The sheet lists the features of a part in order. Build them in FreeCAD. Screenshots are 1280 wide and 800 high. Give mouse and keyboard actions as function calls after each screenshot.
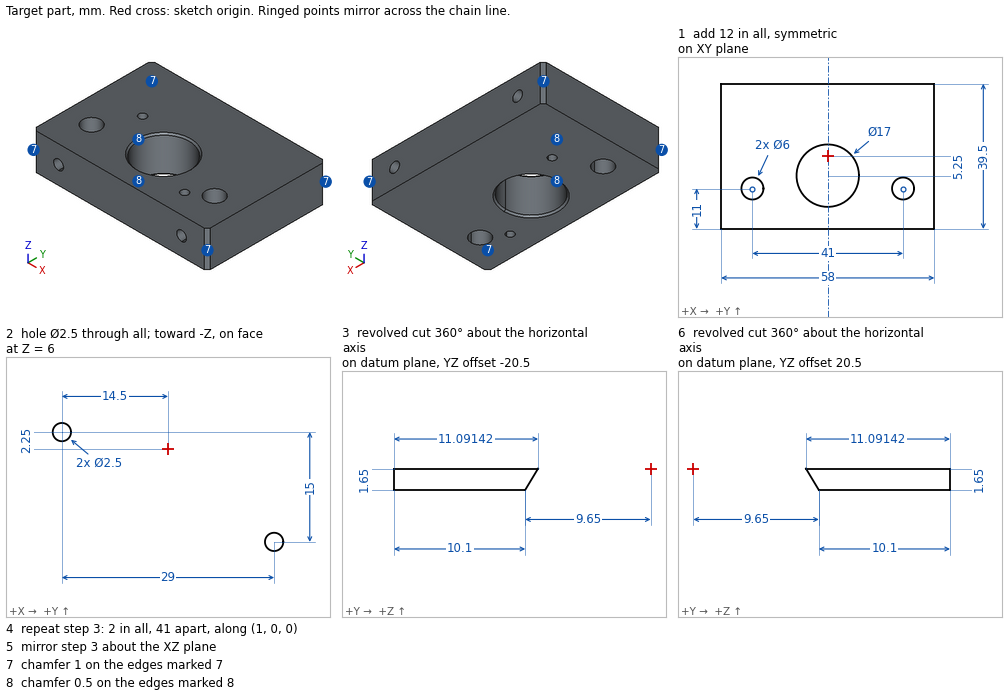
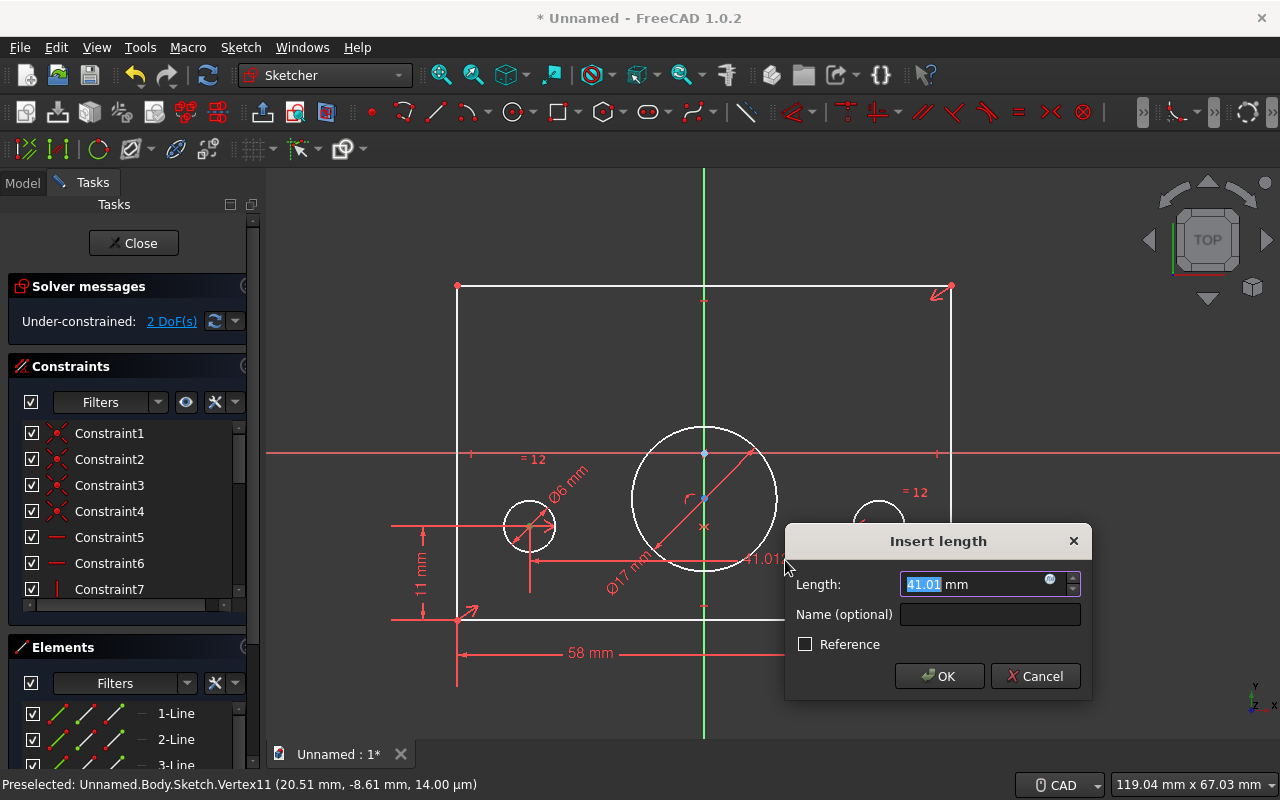
text(41)
key(Return)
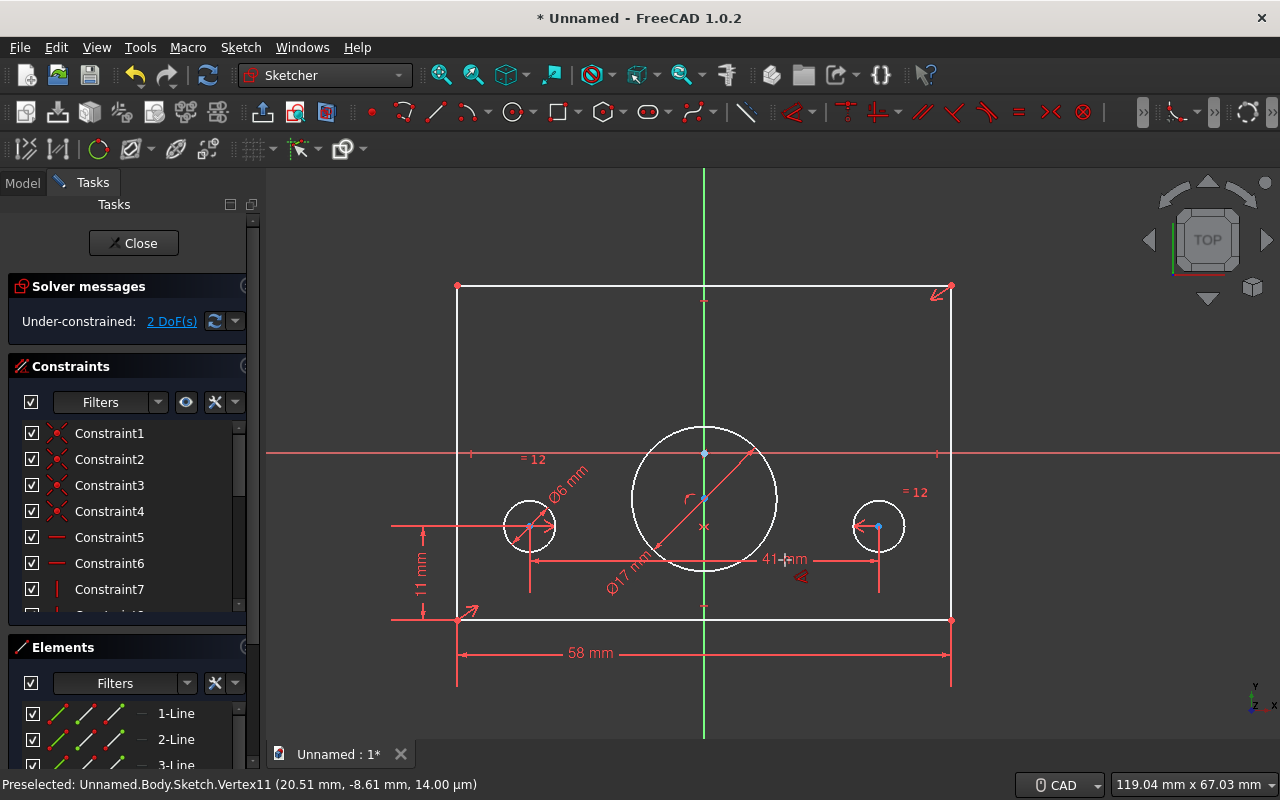
click(951, 520)
click(985, 376)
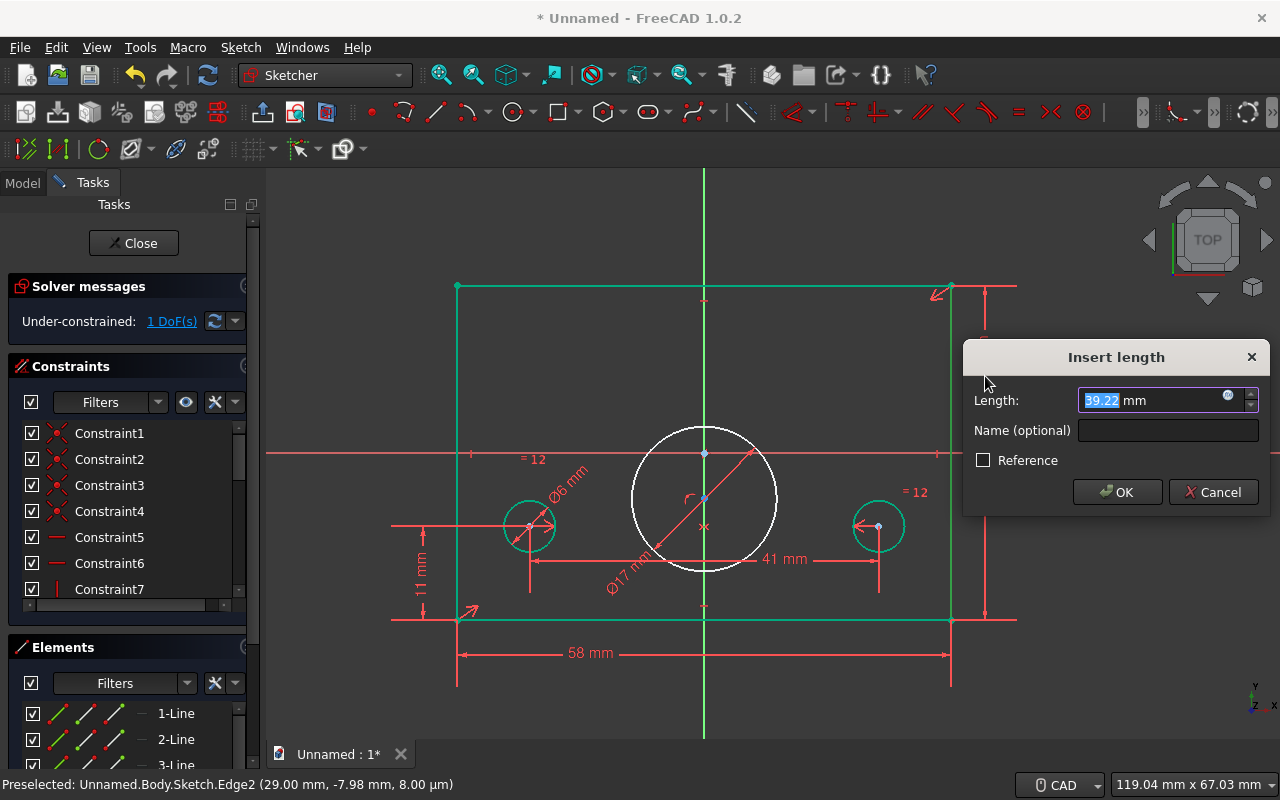
text(39.5)
key(Return)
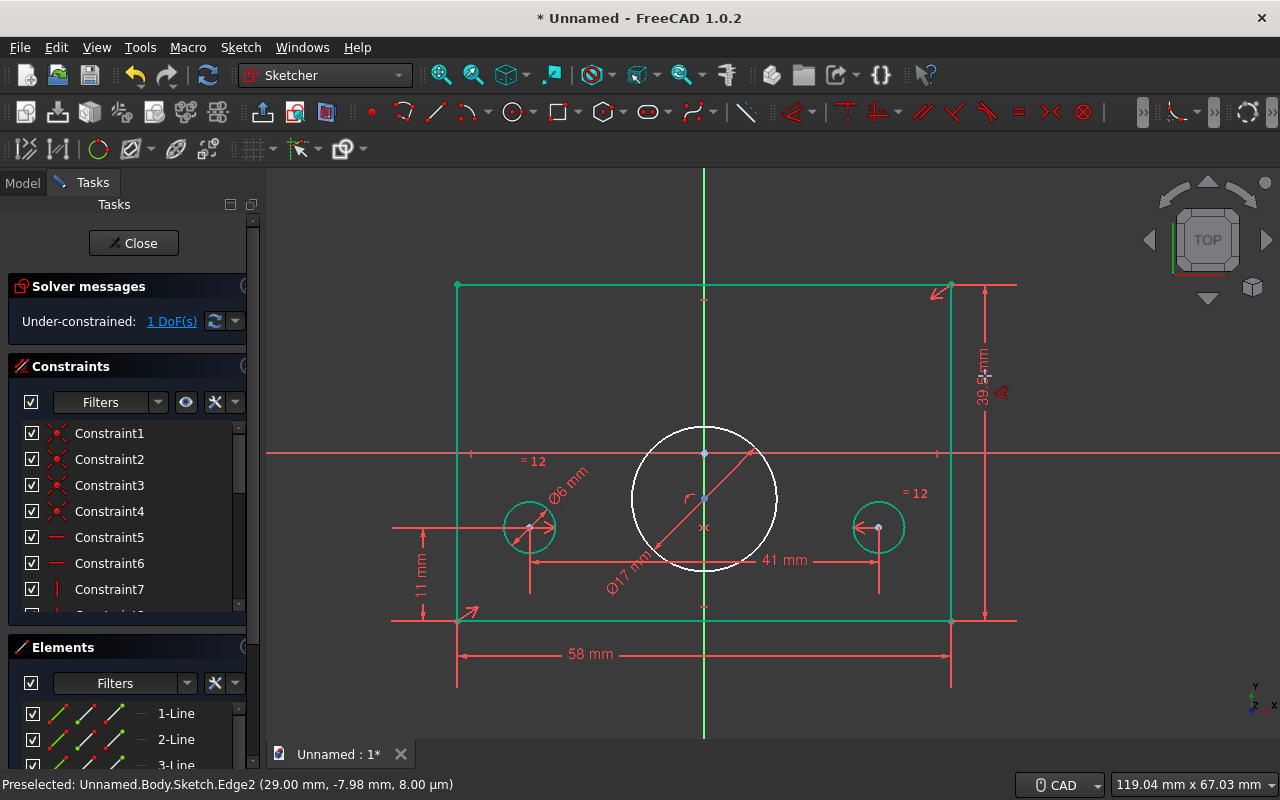
click(704, 499)
click(738, 476)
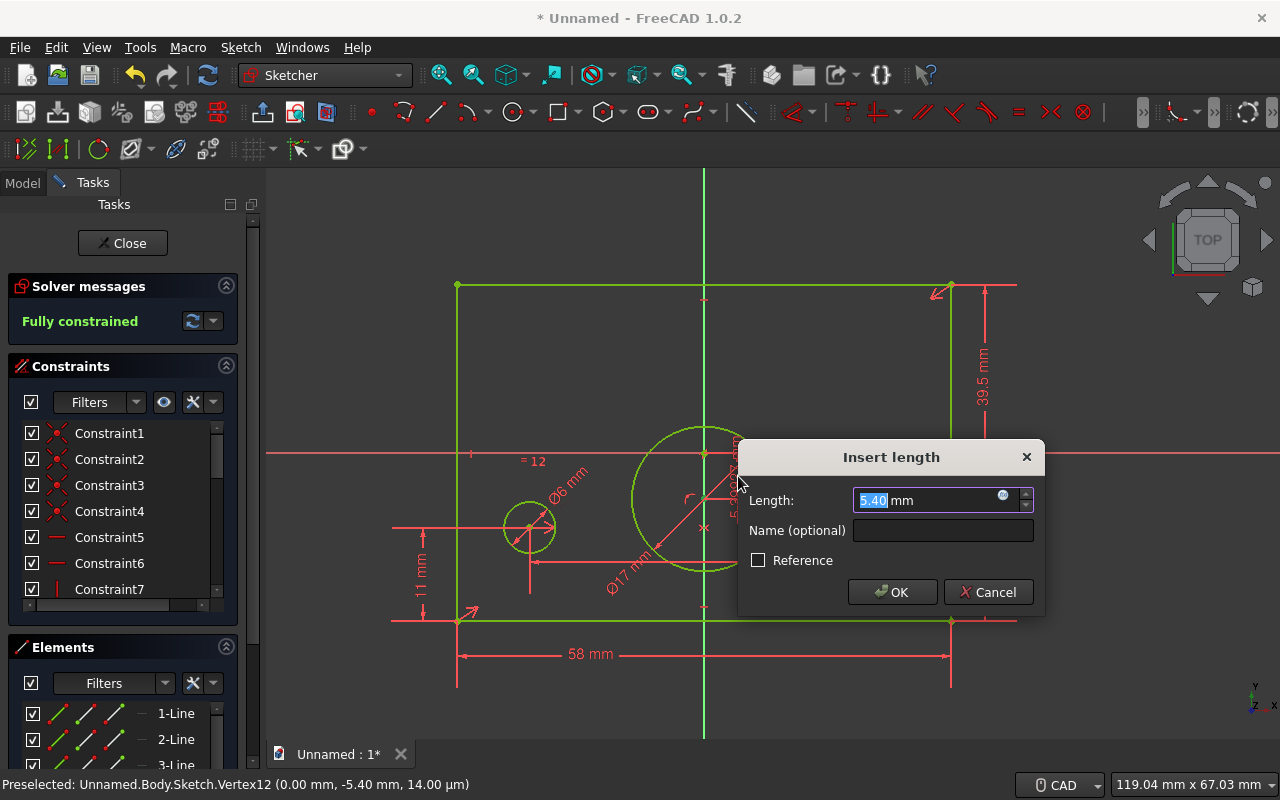
text(5.25)
key(Return)
key(Escape)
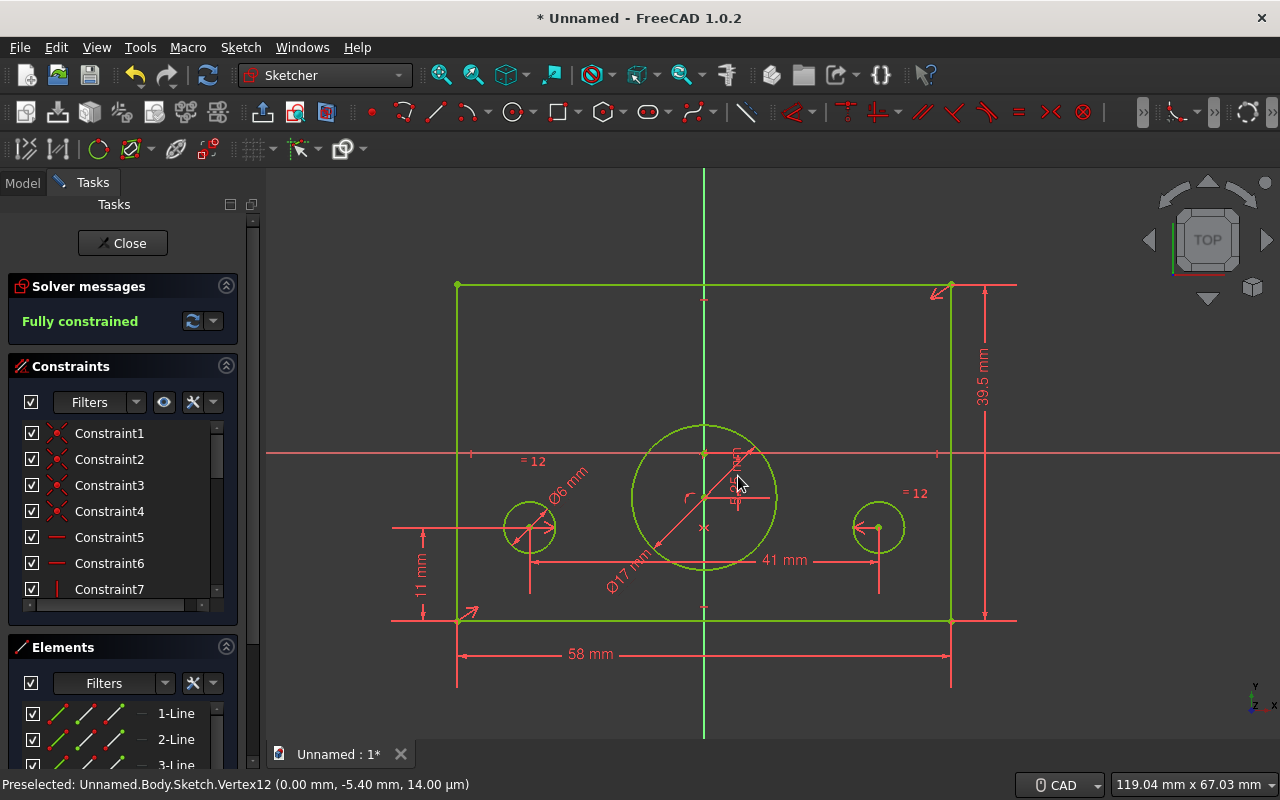
click(123, 243)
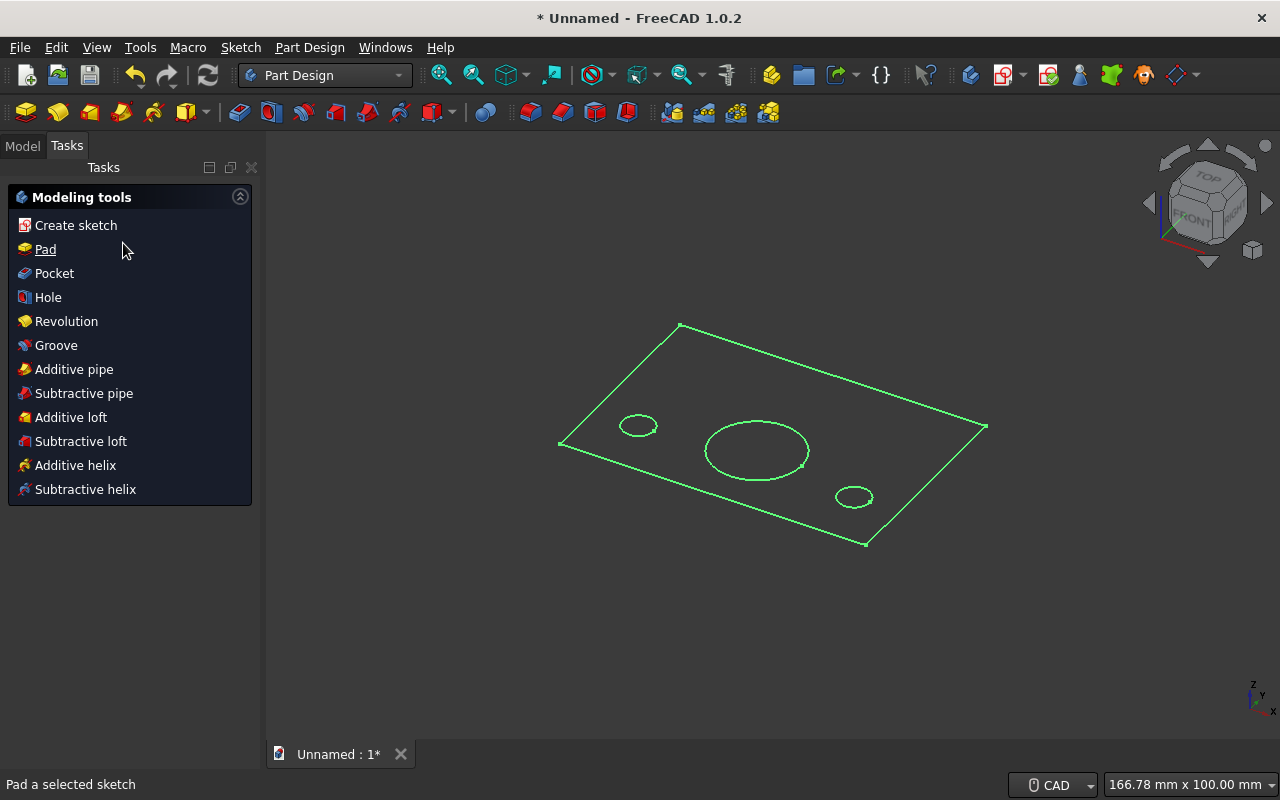
click(26, 112)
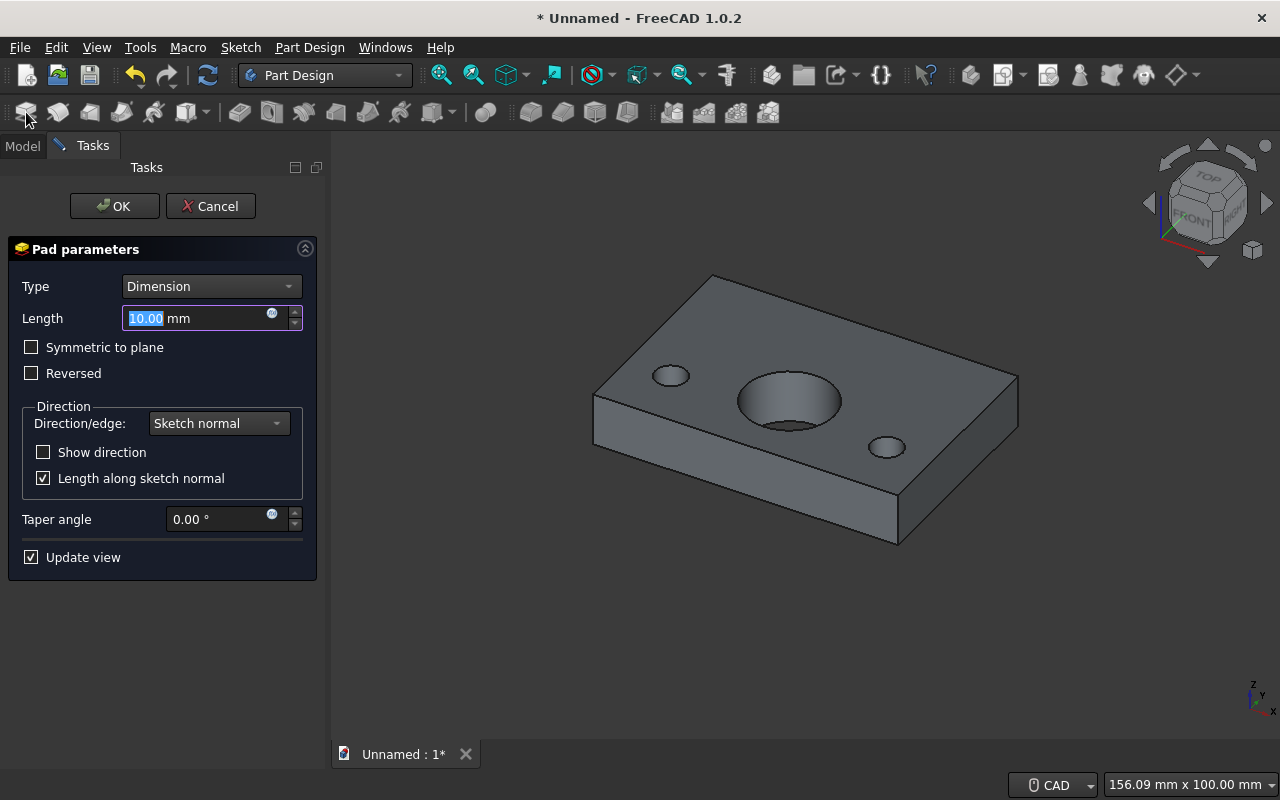
text(12)
key(Tab)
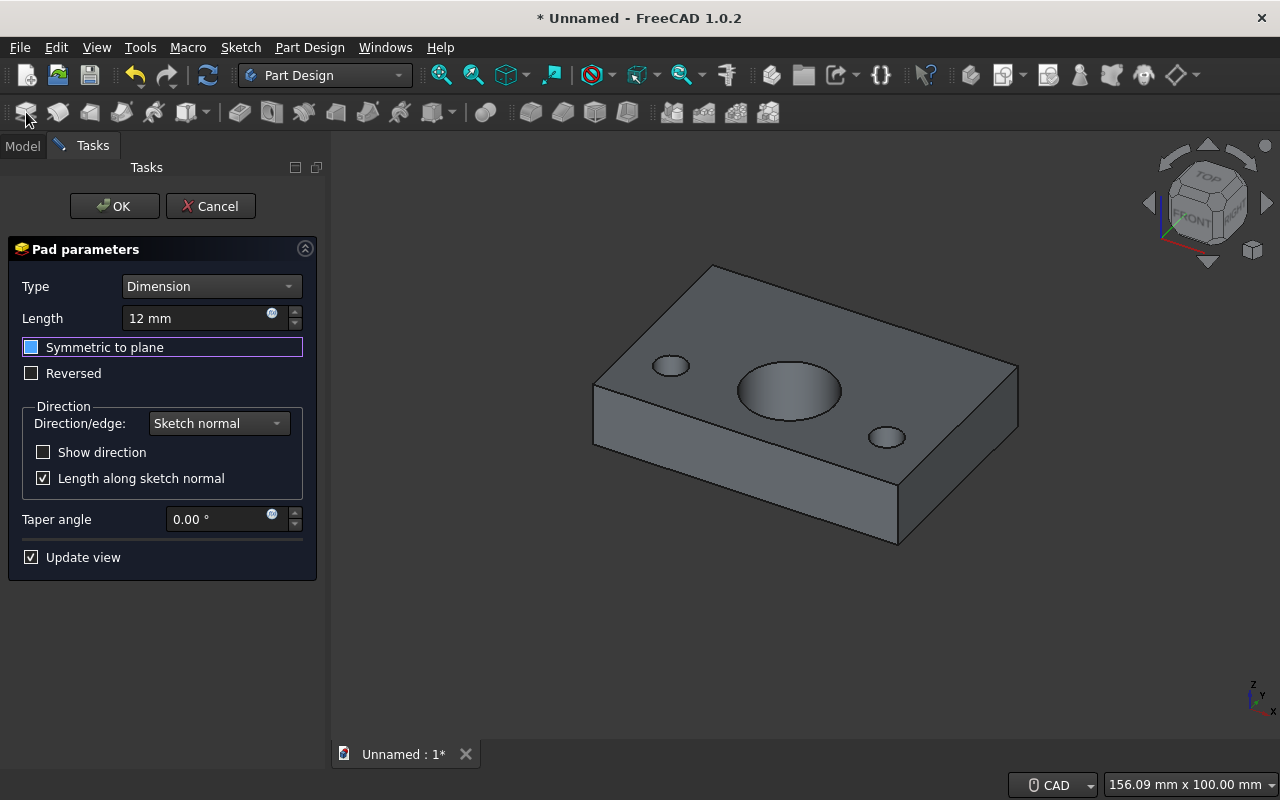
click(30, 347)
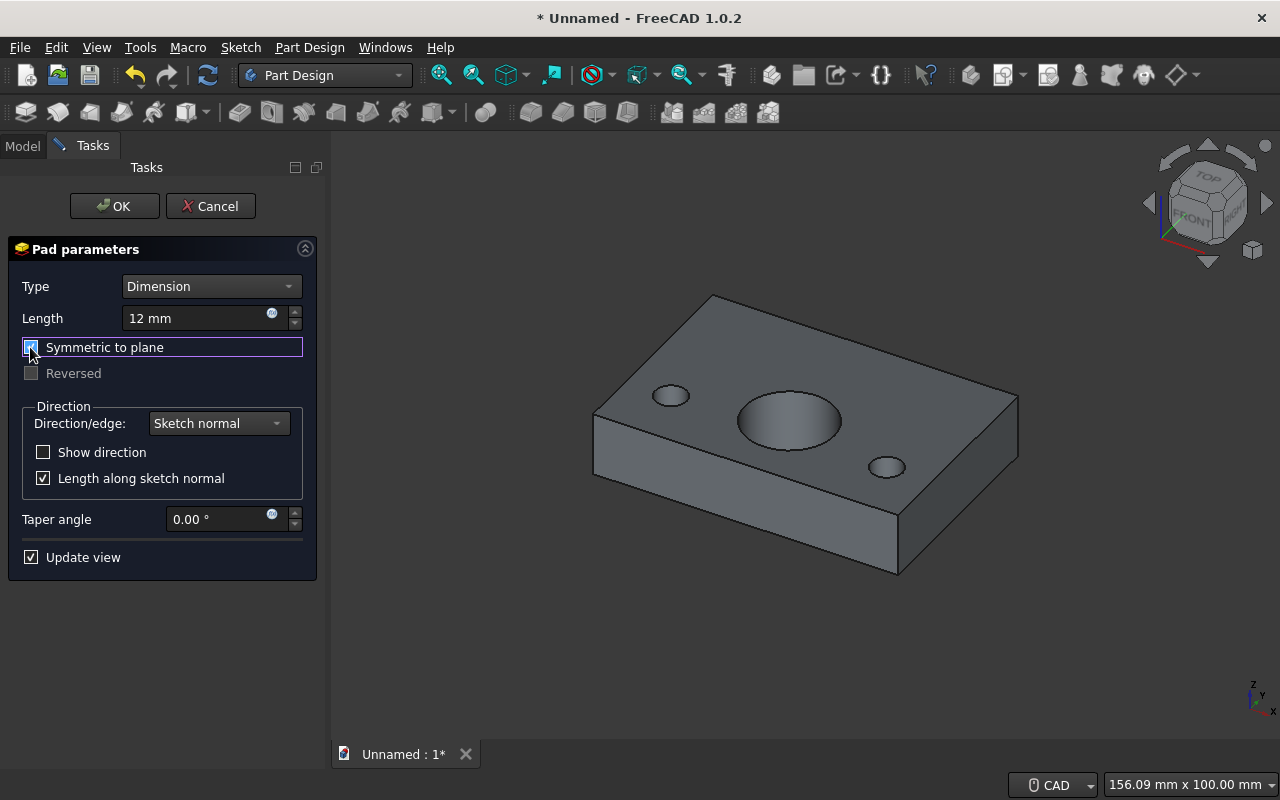
click(115, 206)